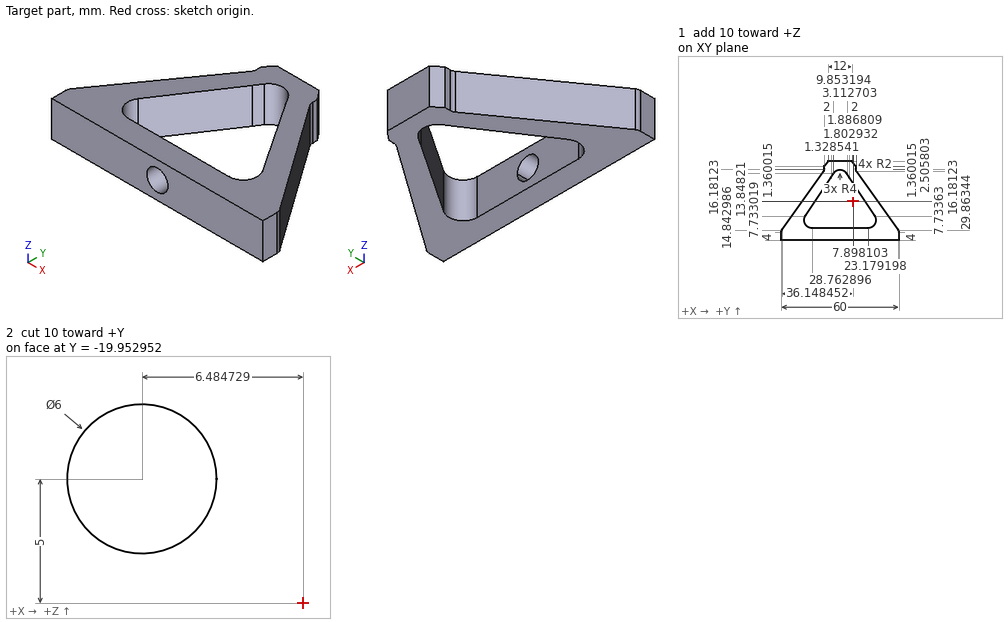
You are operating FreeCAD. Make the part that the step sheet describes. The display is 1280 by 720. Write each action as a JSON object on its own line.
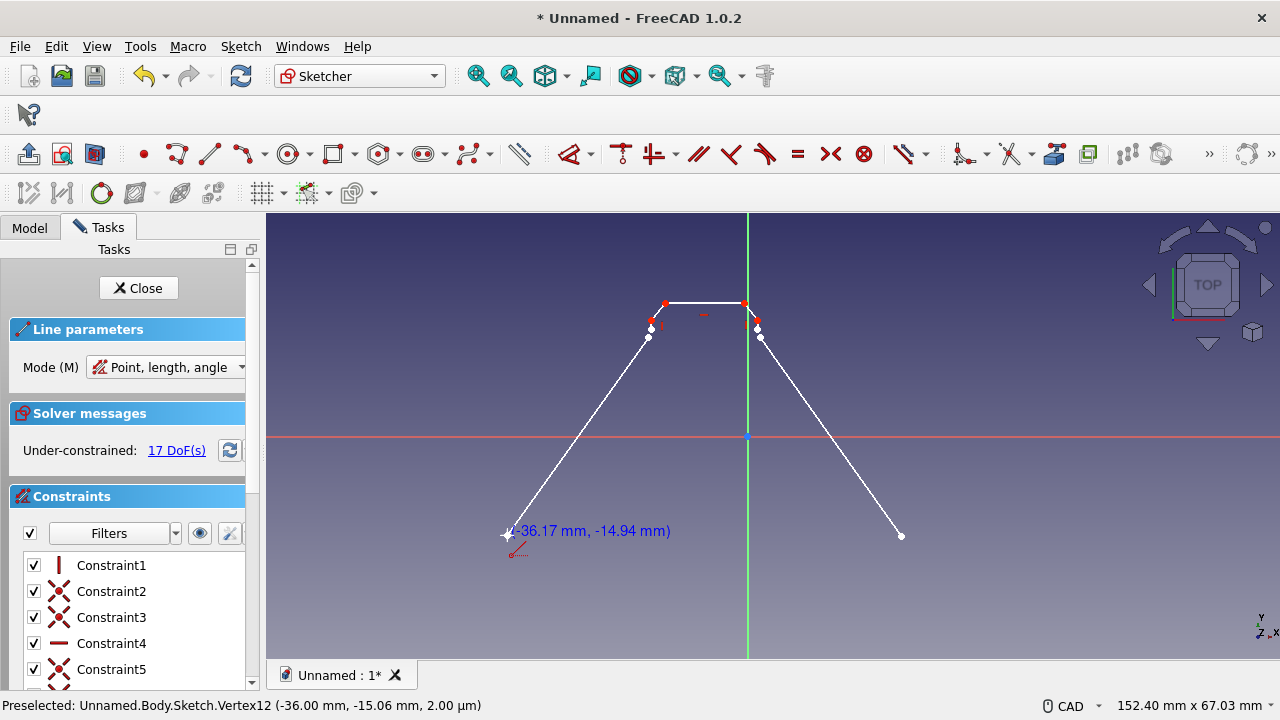
{"action": "left_click", "coordinate": [177, 154]}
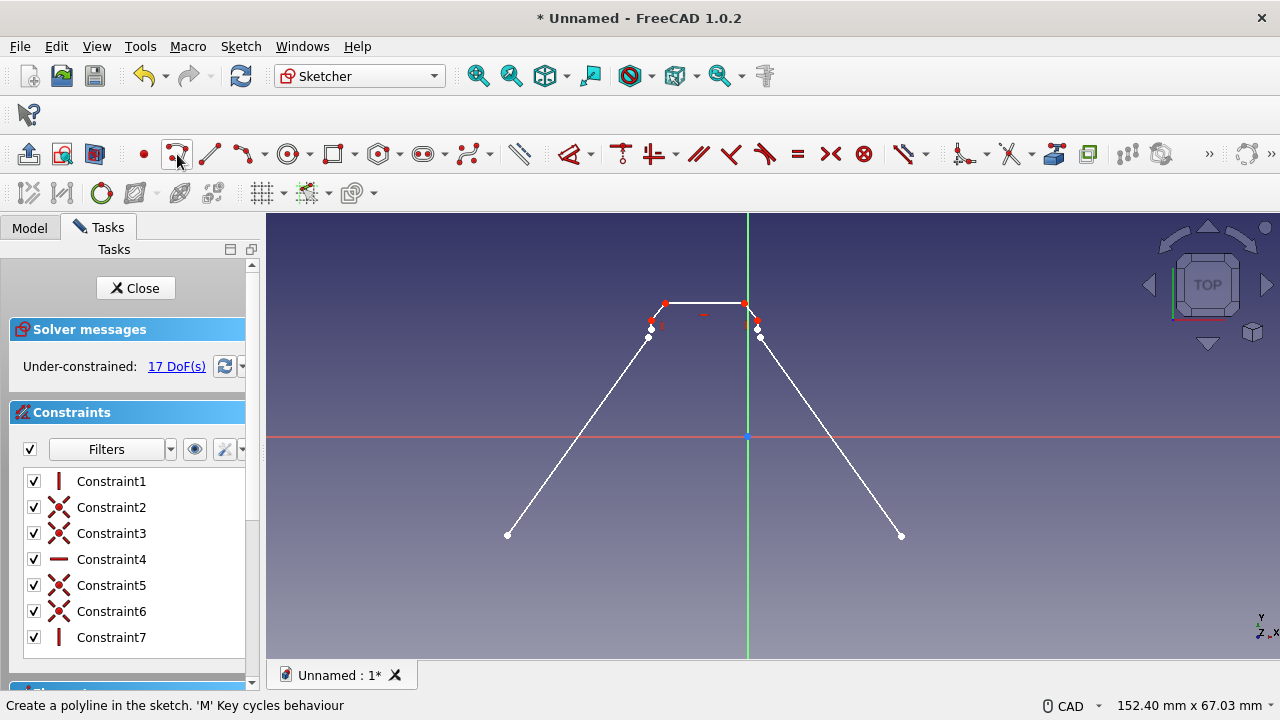
{"action": "scroll", "coordinate": [505, 543], "scroll_direction": "up", "scroll_amount": 4}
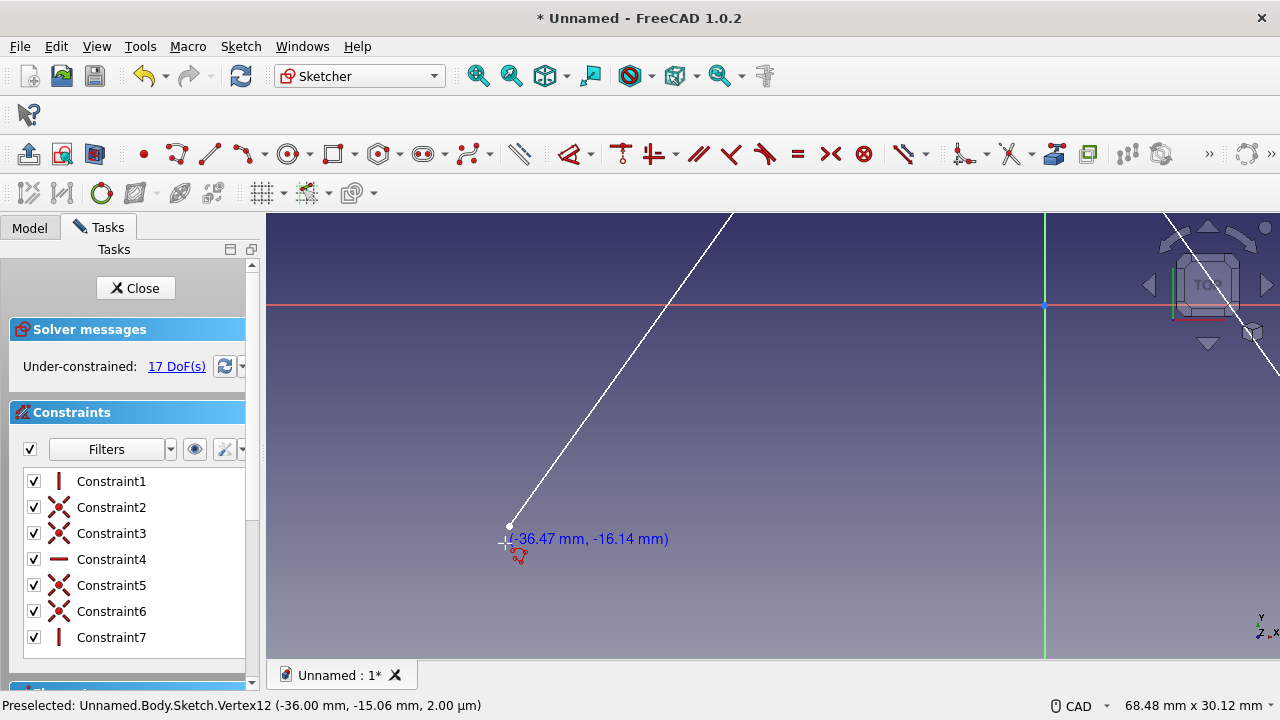
{"action": "left_click", "coordinate": [505, 542]}
{"action": "left_click", "coordinate": [505, 601]}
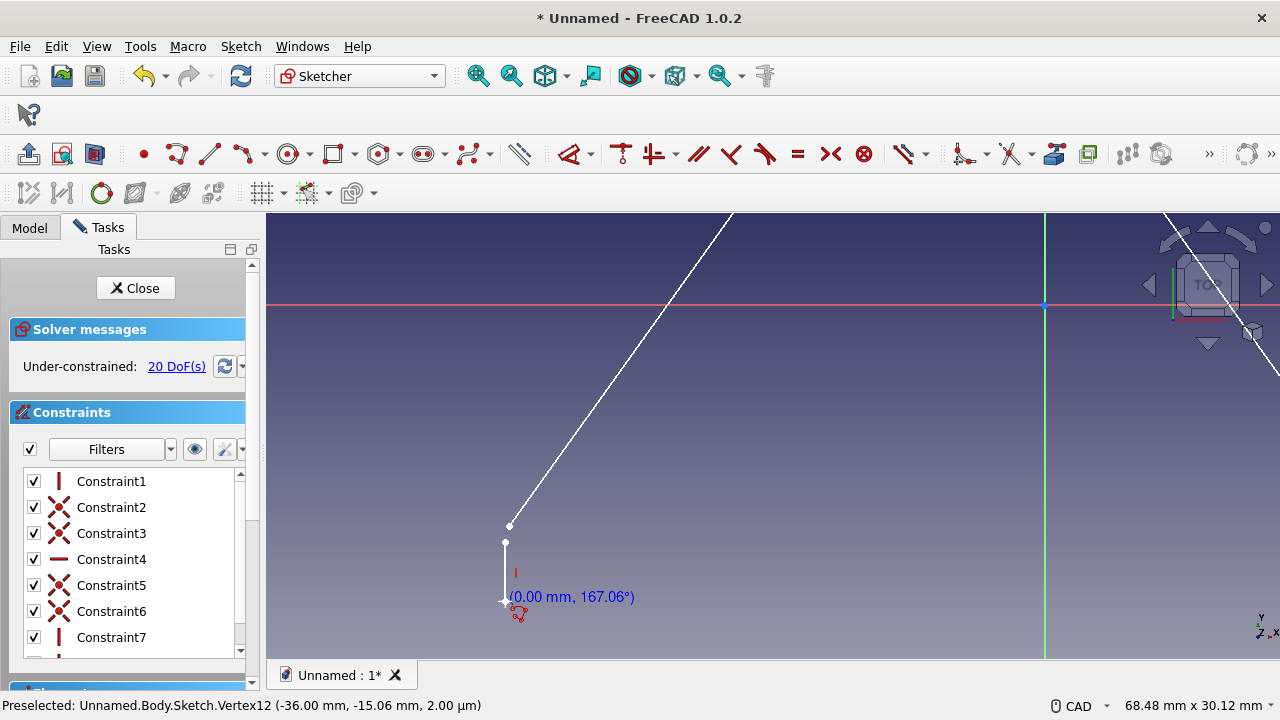
{"action": "scroll", "coordinate": [505, 543], "scroll_direction": "down", "scroll_amount": 4}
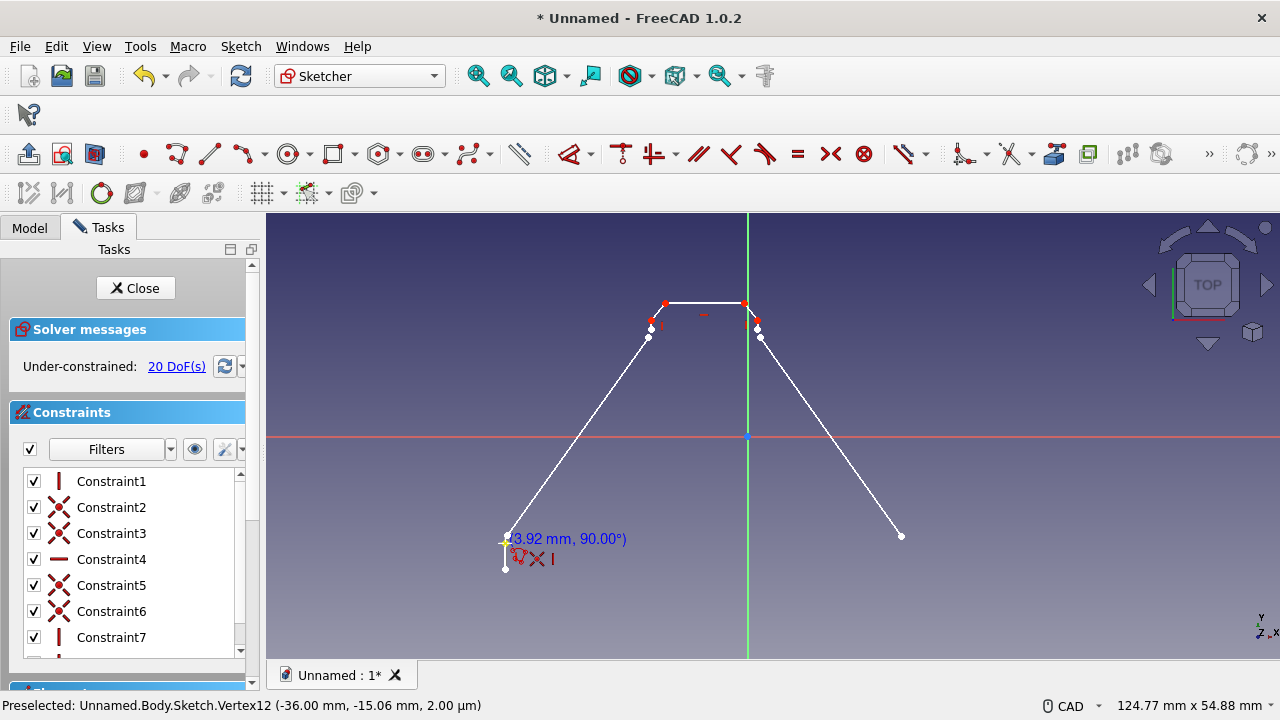
{"action": "left_click", "coordinate": [904, 569]}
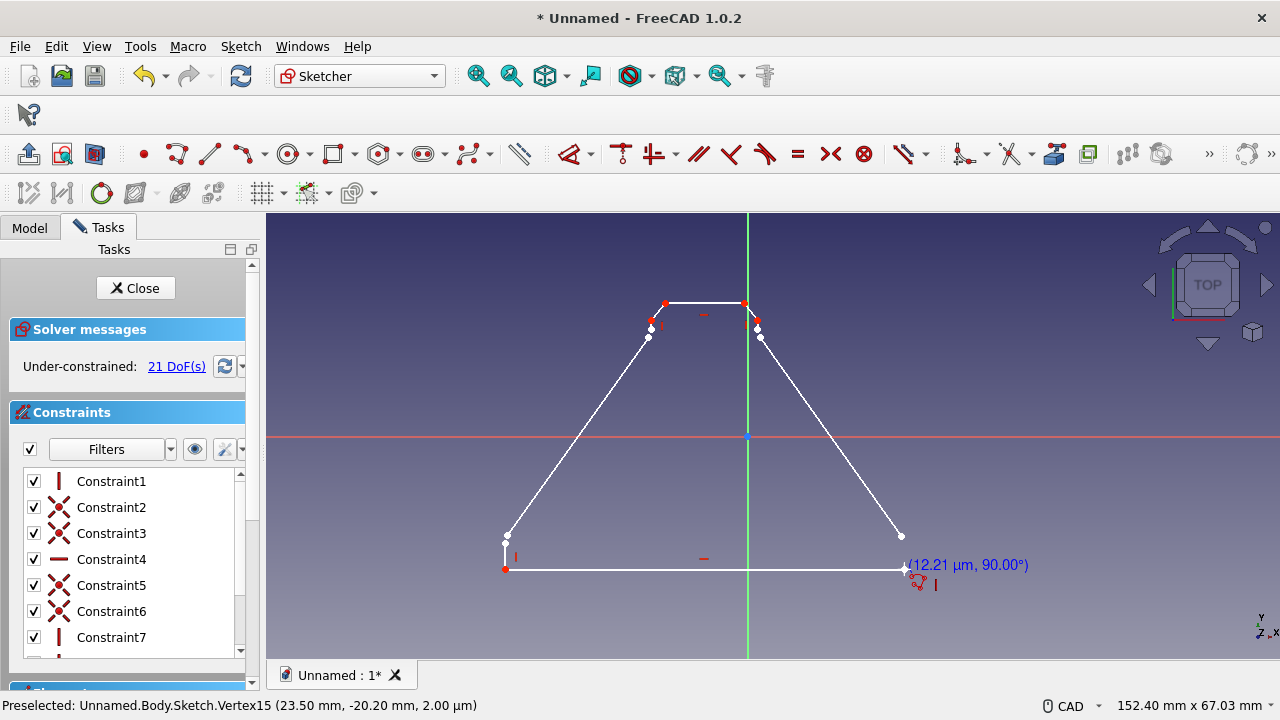
{"action": "scroll", "coordinate": [904, 543], "scroll_direction": "up", "scroll_amount": 4}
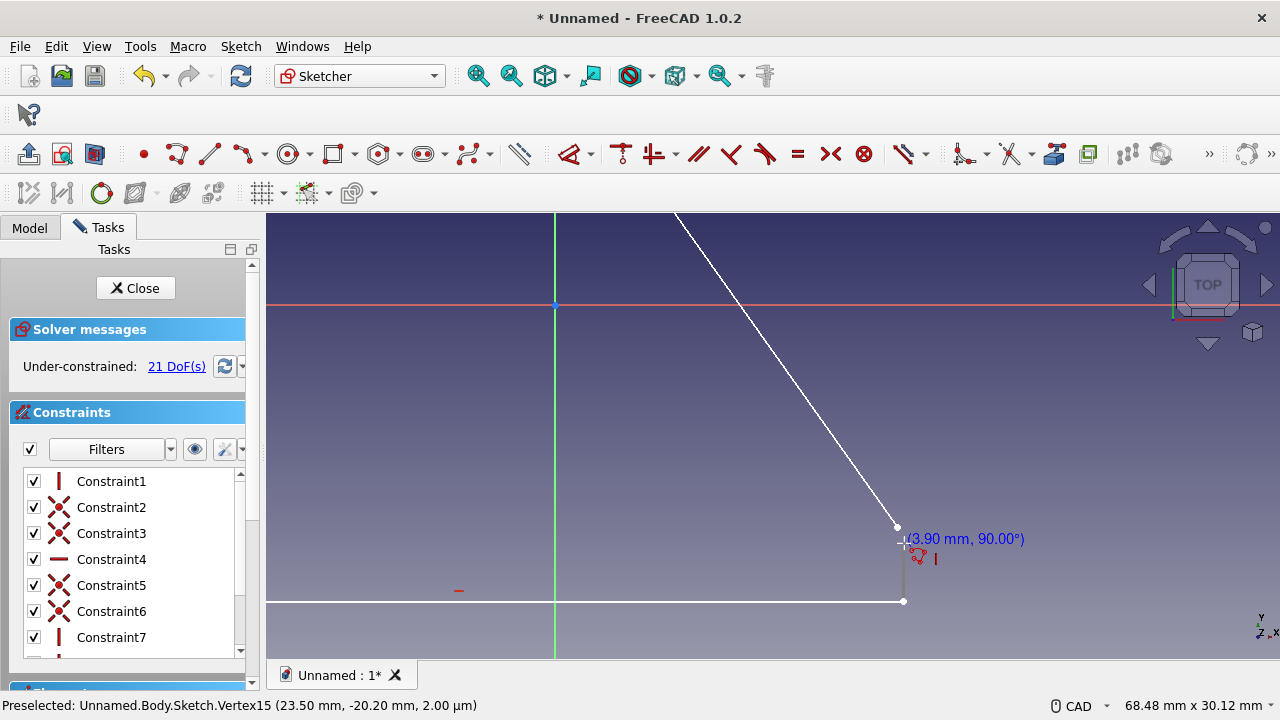
{"action": "left_click", "coordinate": [903, 542]}
{"action": "right_click", "coordinate": [903, 542]}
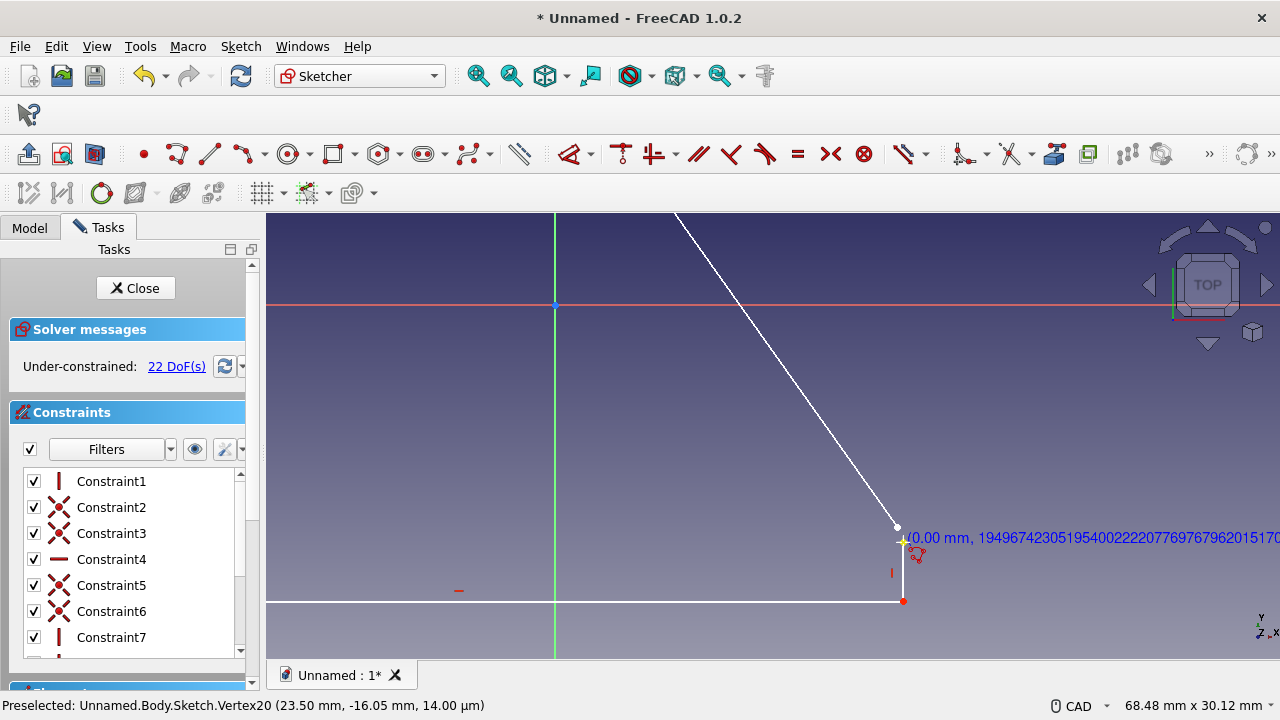
{"action": "left_click", "coordinate": [242, 154]}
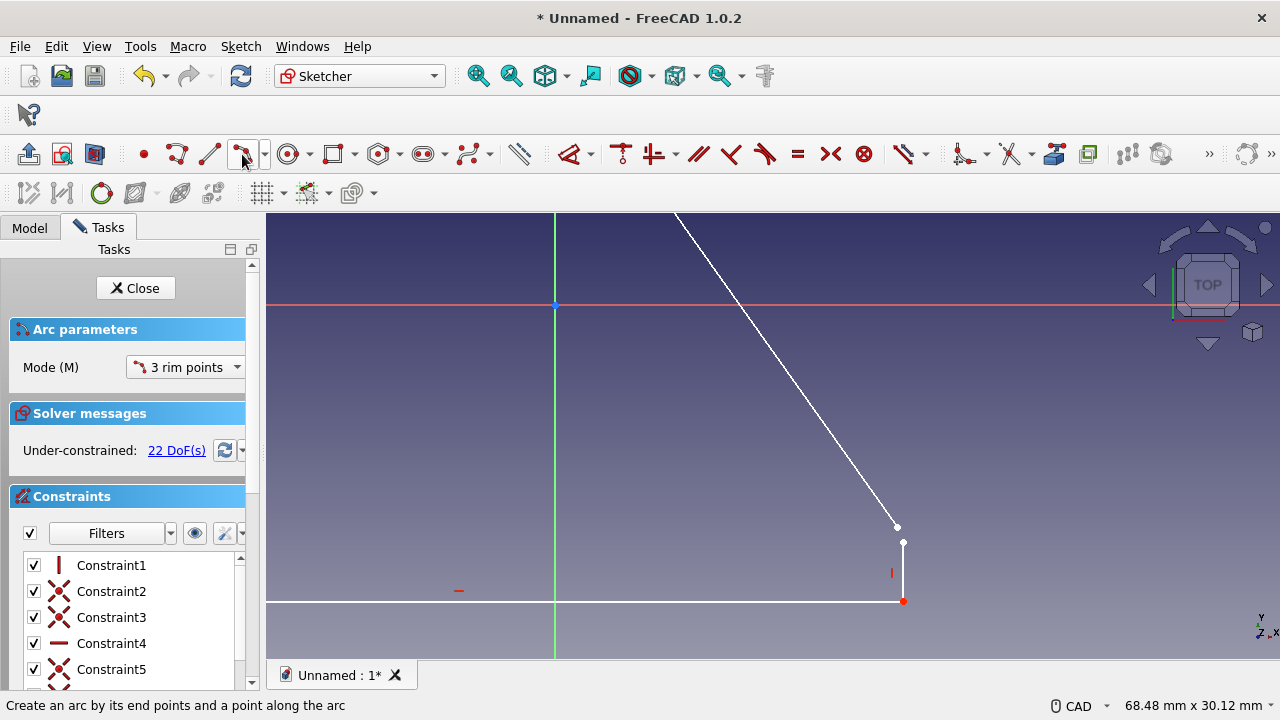
{"action": "scroll", "coordinate": [905, 543], "scroll_direction": "down", "scroll_amount": 4}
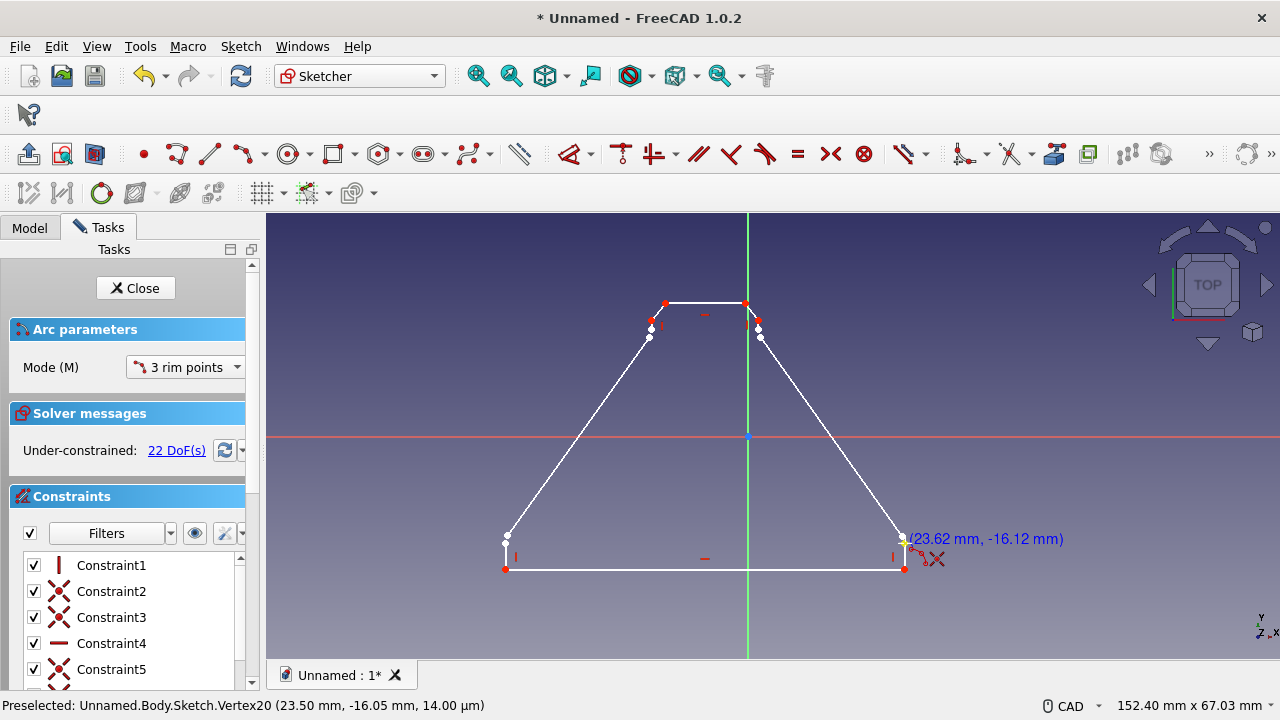
{"action": "scroll", "coordinate": [761, 337], "scroll_direction": "up", "scroll_amount": 4}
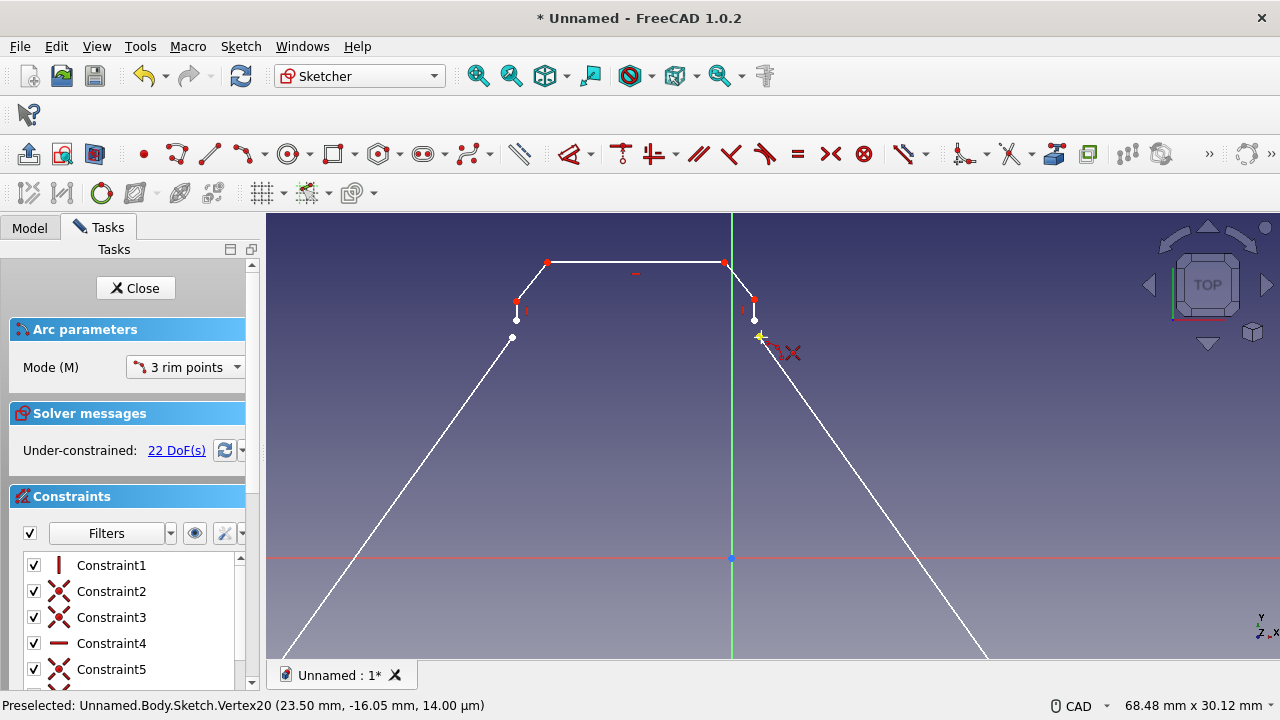
{"action": "left_click", "coordinate": [759, 337]}